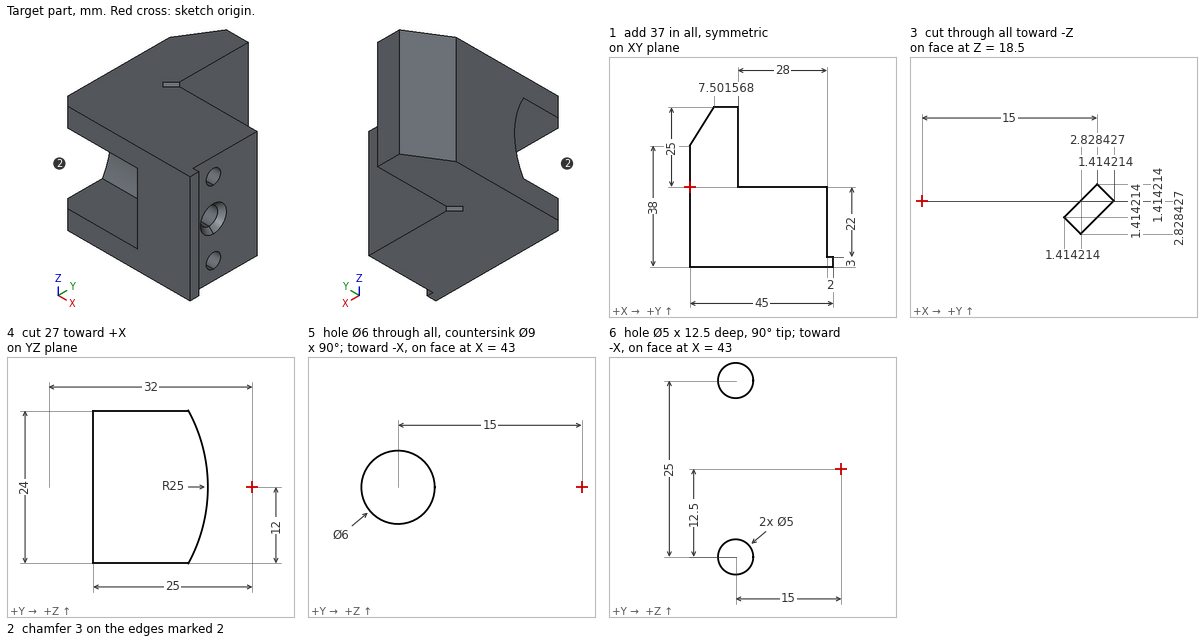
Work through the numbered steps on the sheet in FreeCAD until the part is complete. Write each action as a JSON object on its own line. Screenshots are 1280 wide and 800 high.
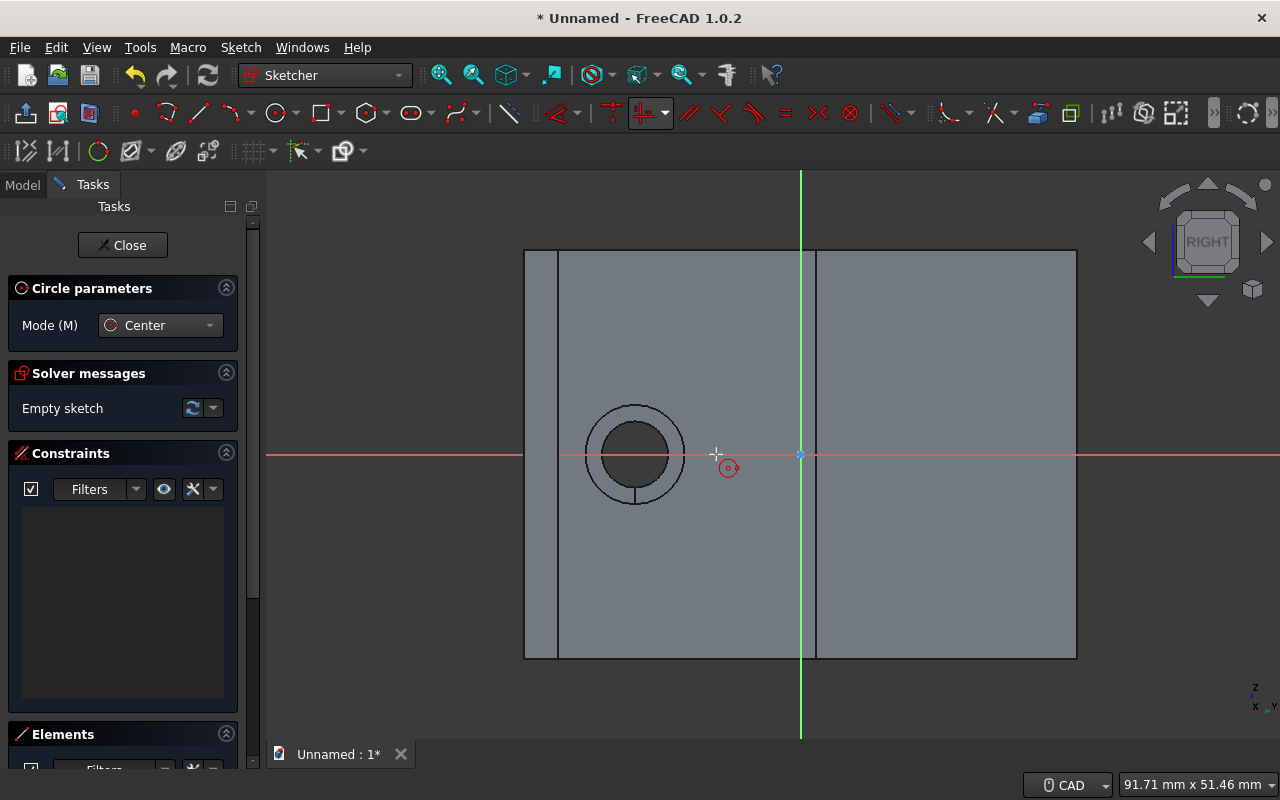
{"action": "left_click", "coordinate": [635, 593]}
{"action": "left_click", "coordinate": [655, 573]}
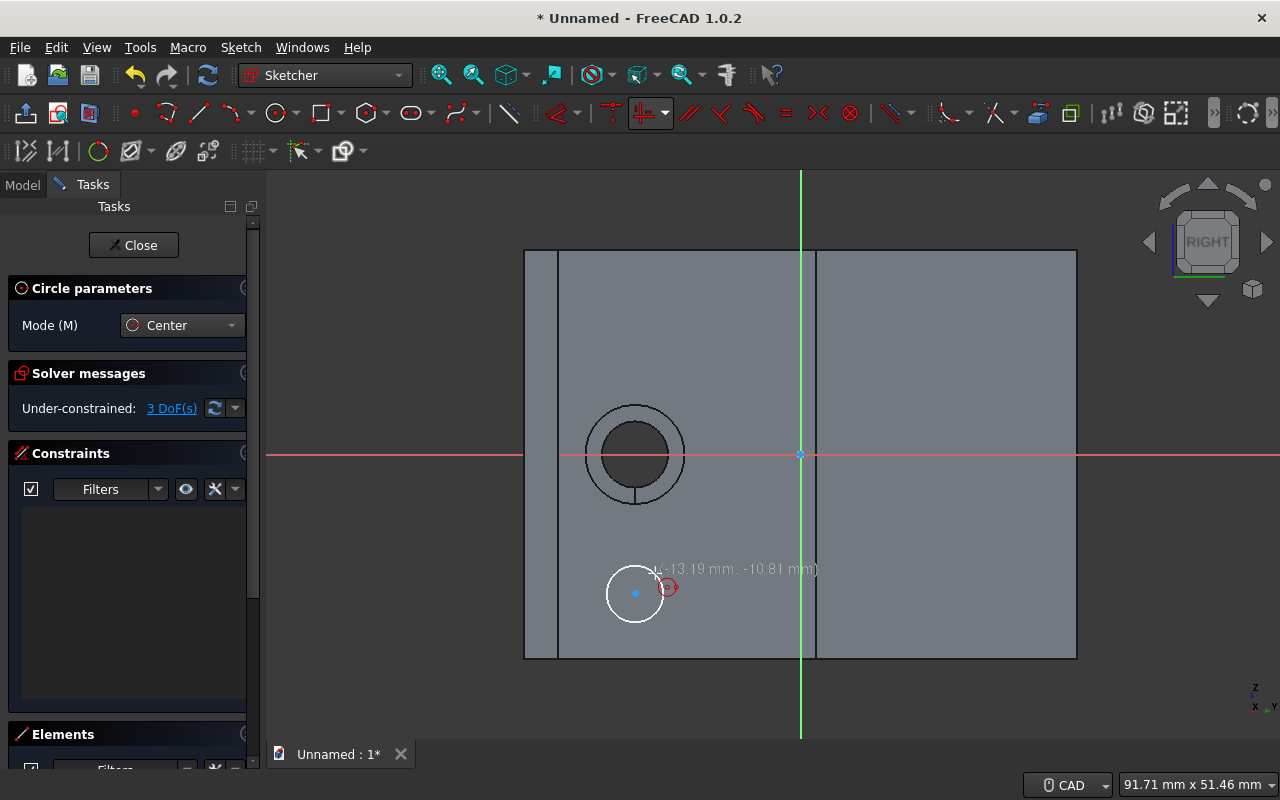
{"action": "left_click", "coordinate": [635, 316]}
{"action": "left_click", "coordinate": [655, 297]}
{"action": "key", "text": "Escape"}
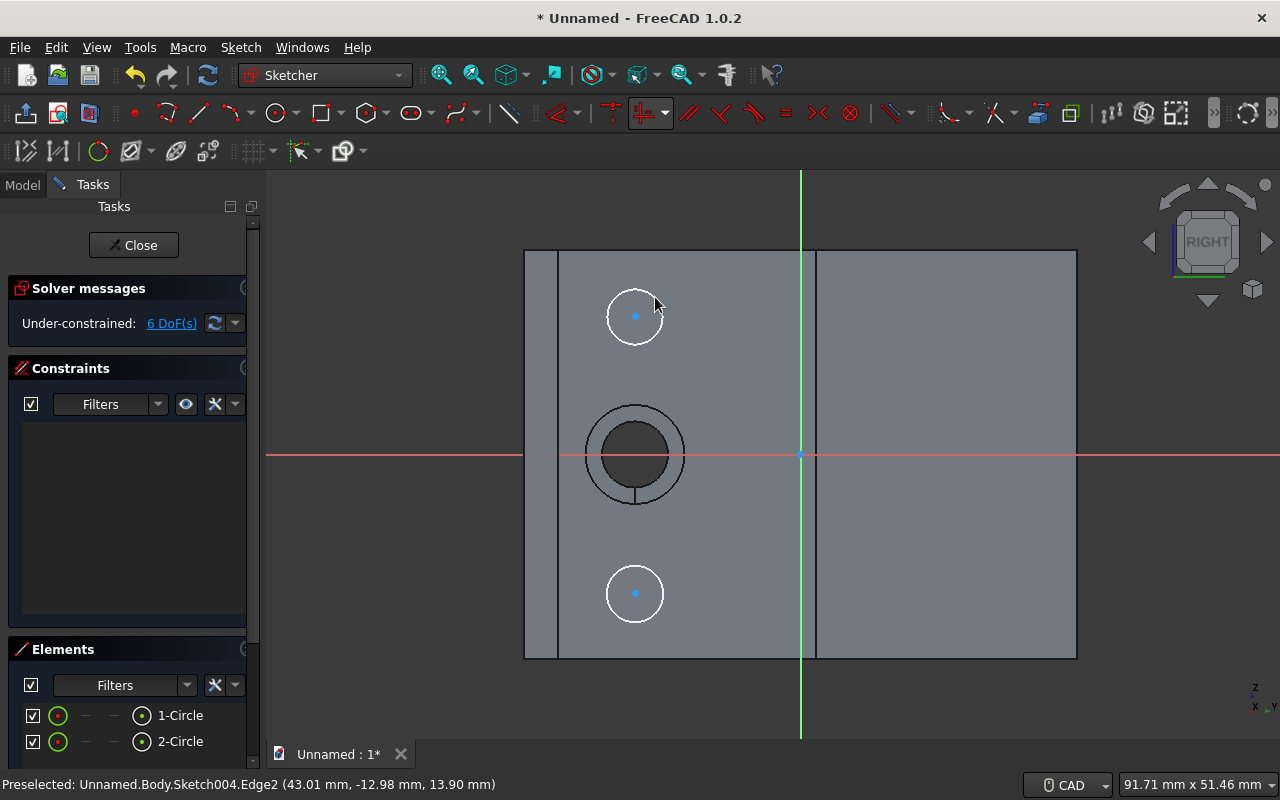
{"action": "left_click", "coordinate": [655, 574]}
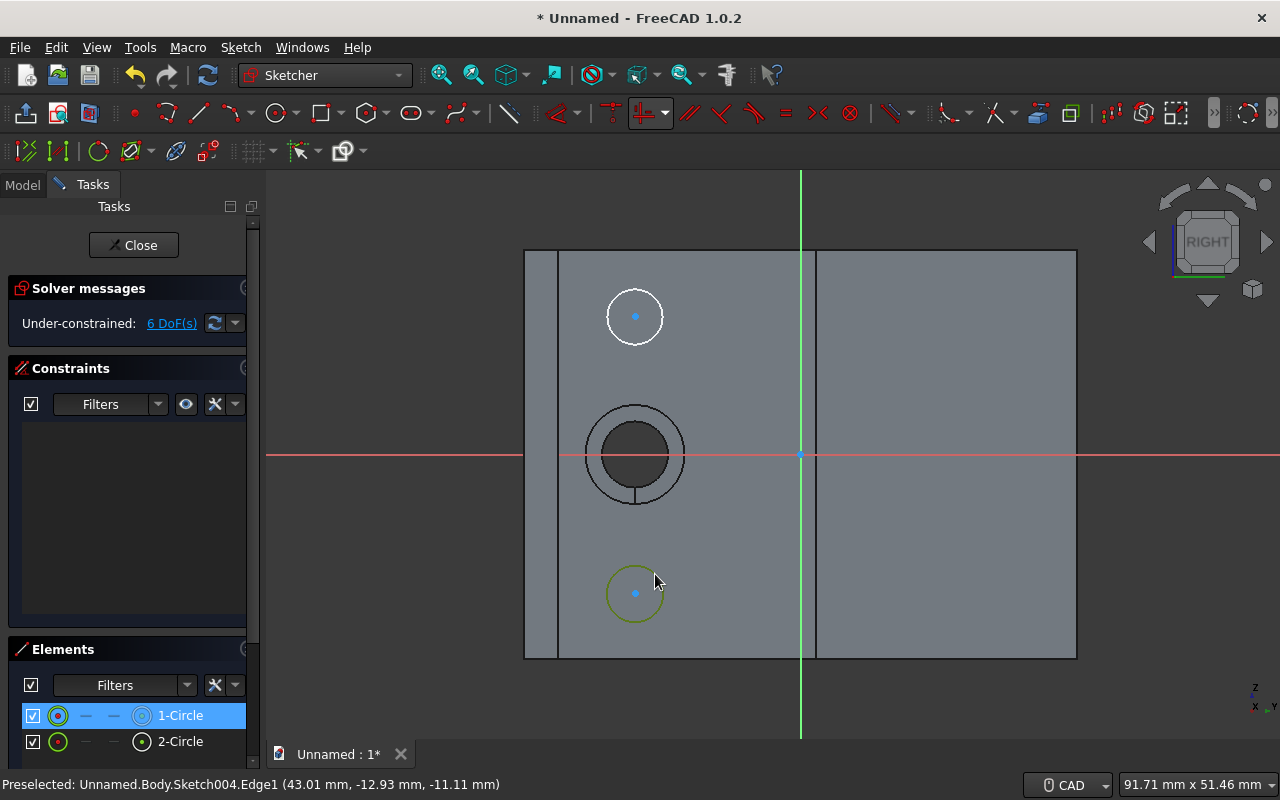
{"action": "left_click", "coordinate": [654, 297]}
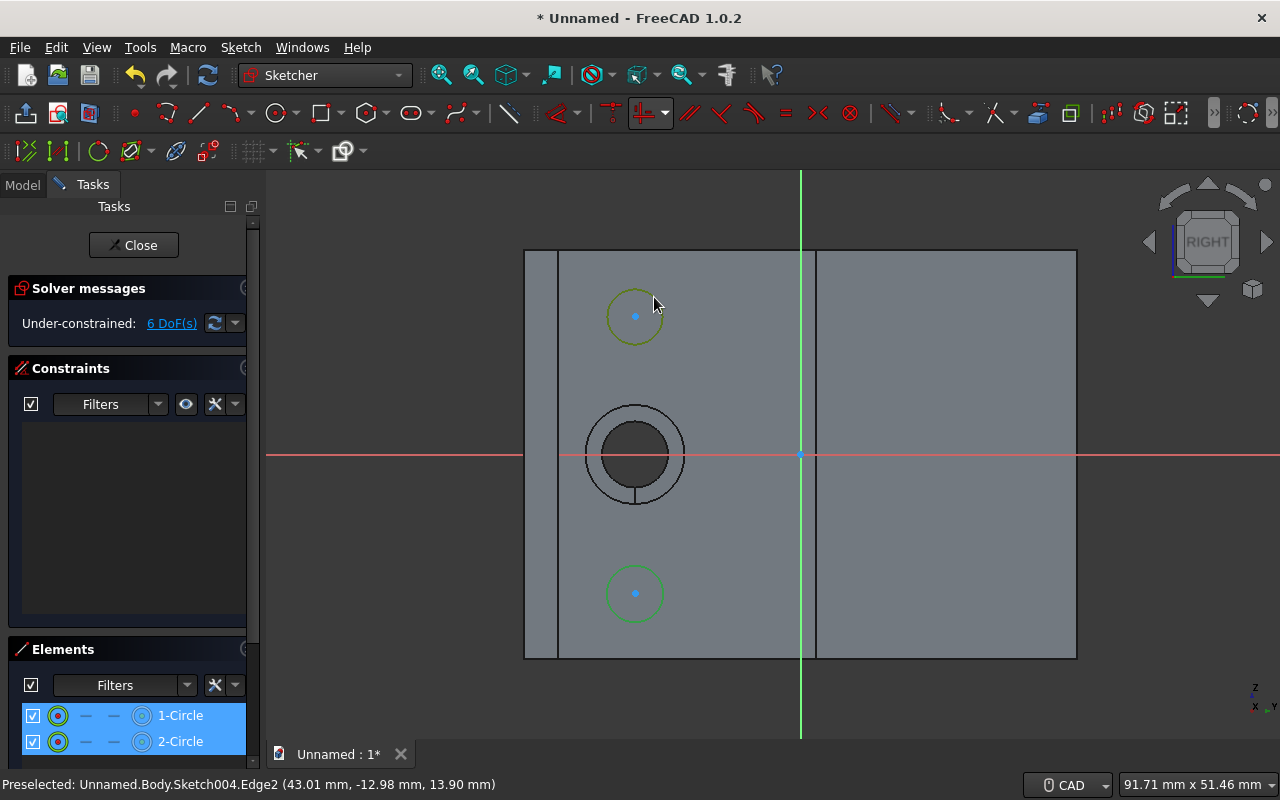
{"action": "key", "text": "e"}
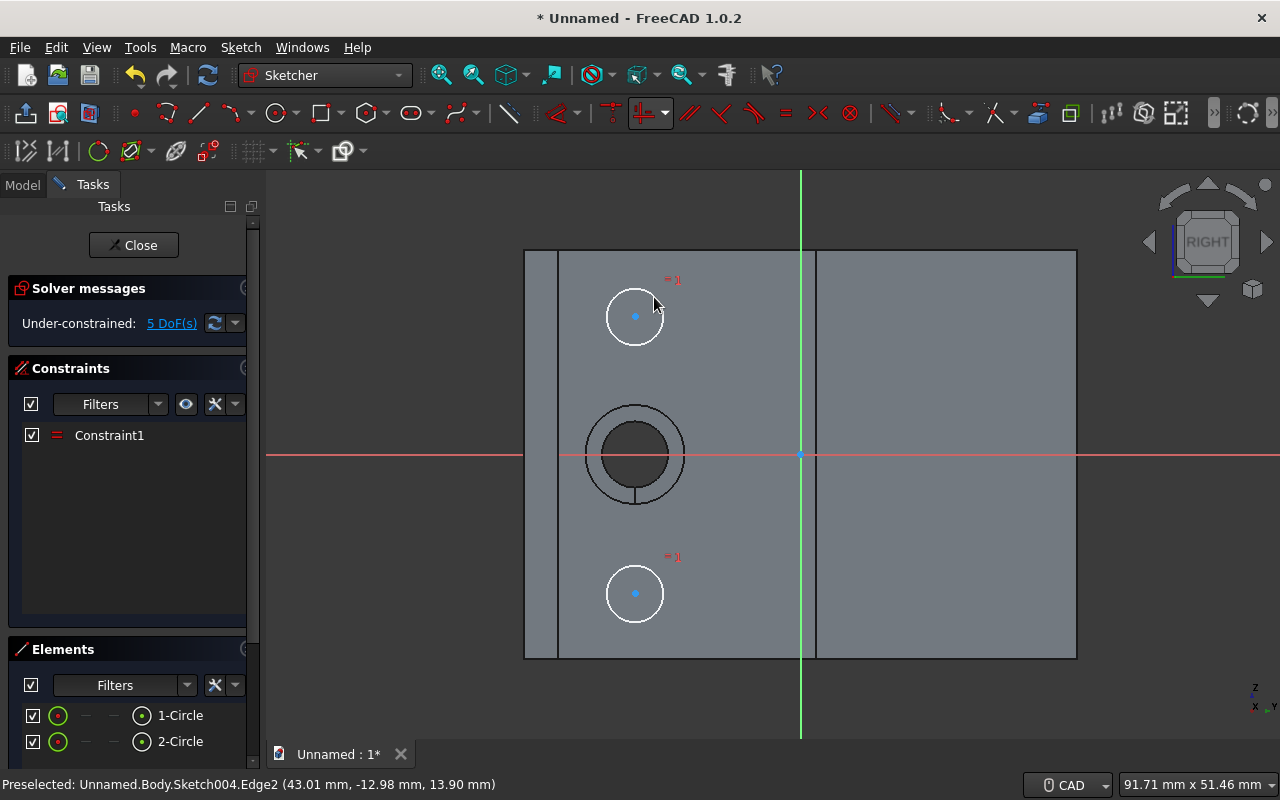
{"action": "left_click", "coordinate": [635, 594]}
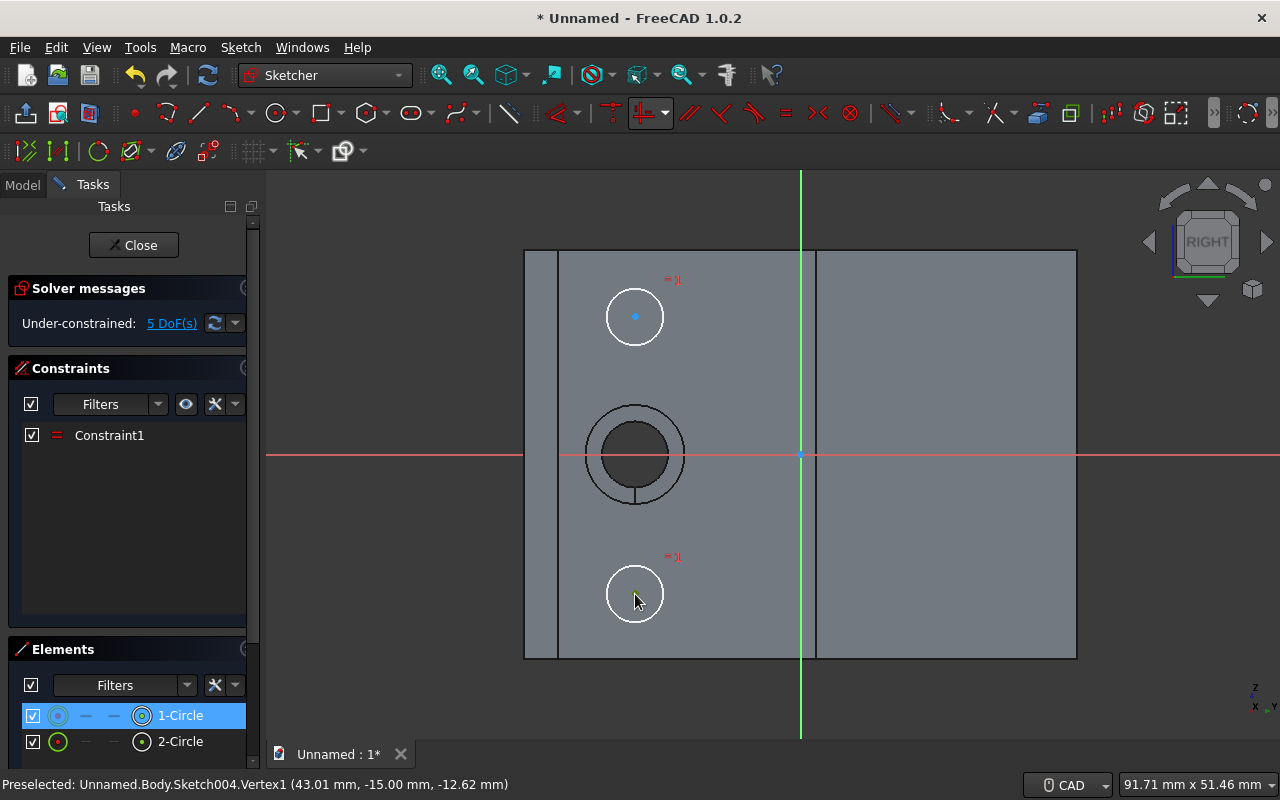
{"action": "left_click", "coordinate": [635, 317]}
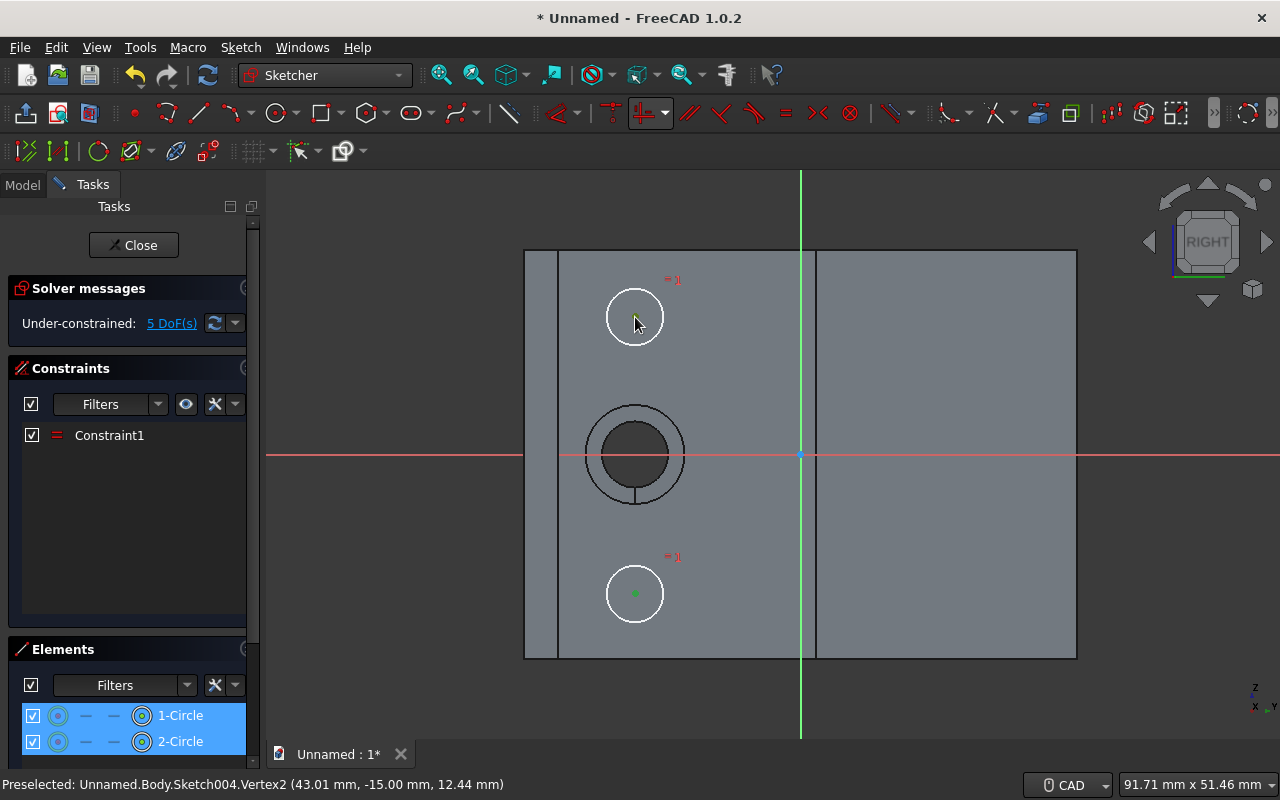
{"action": "left_click", "coordinate": [668, 114]}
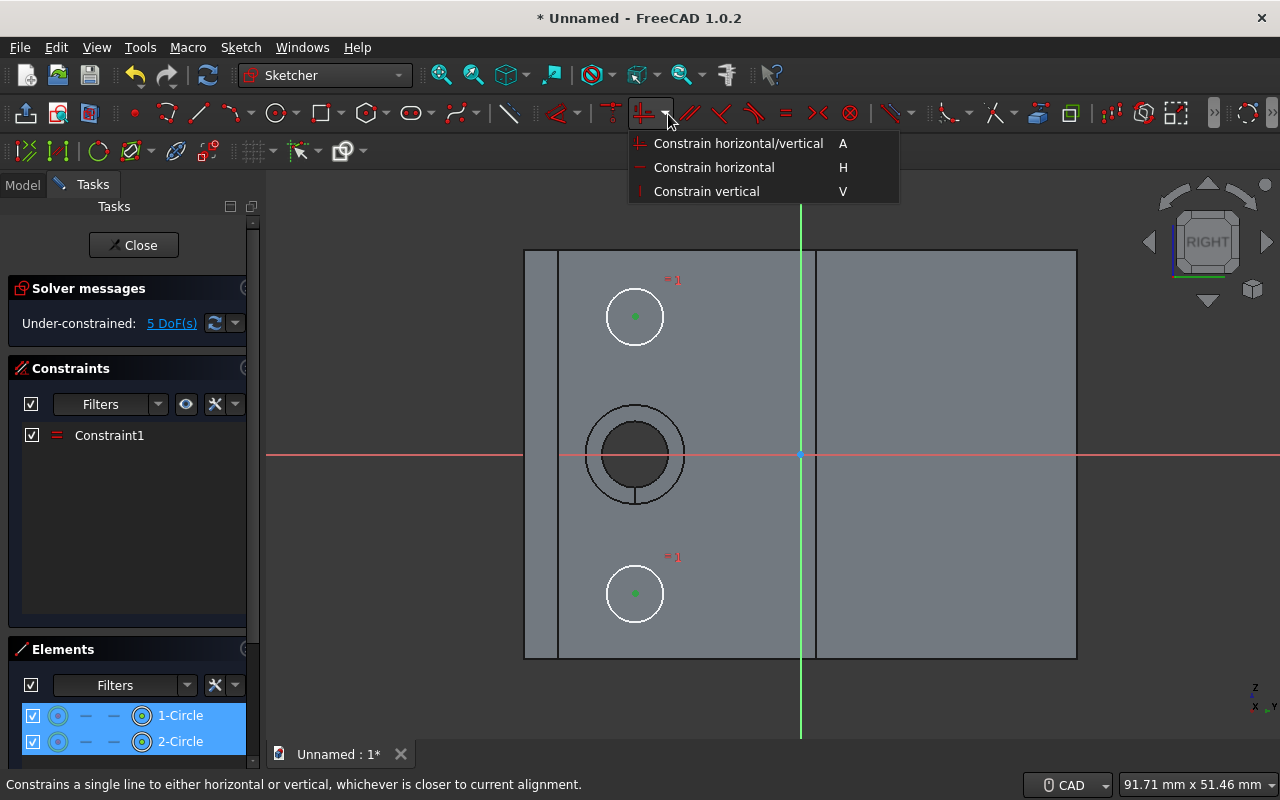
{"action": "left_click", "coordinate": [764, 191]}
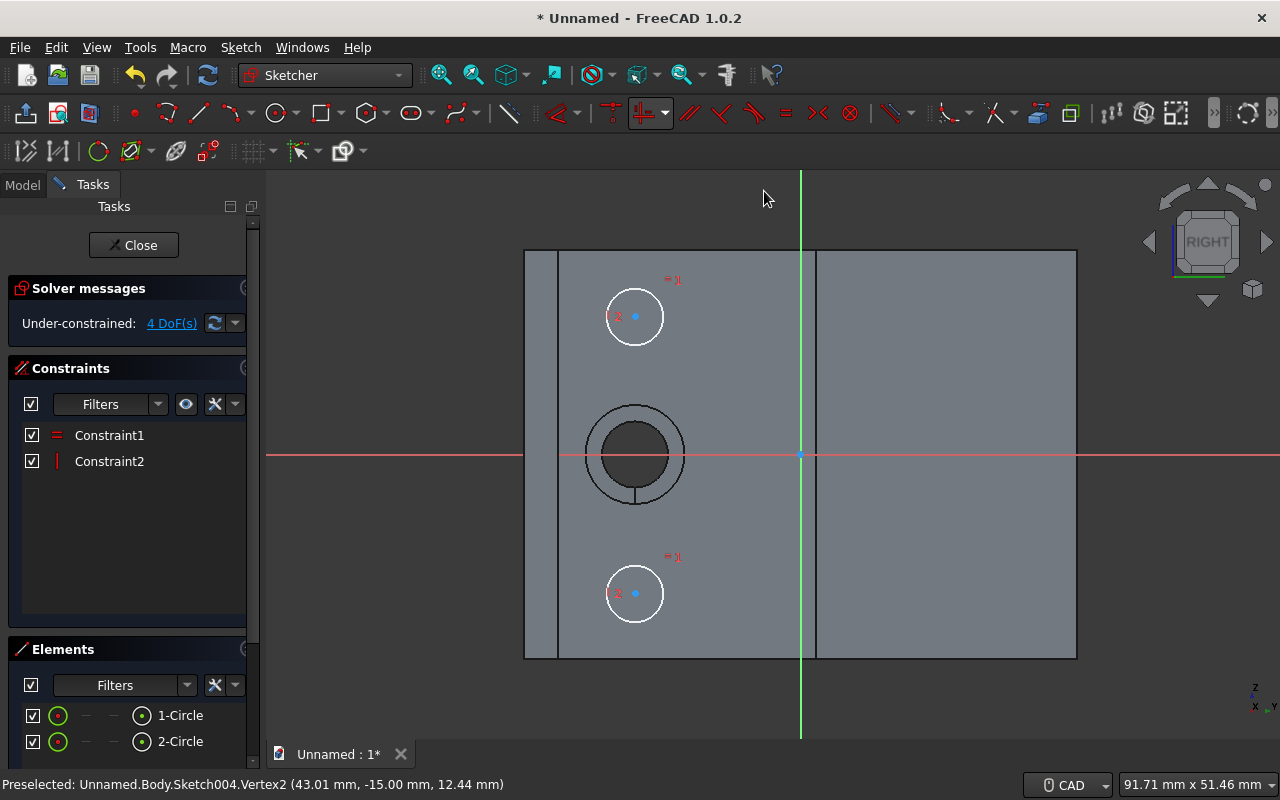
{"action": "left_click", "coordinate": [556, 114]}